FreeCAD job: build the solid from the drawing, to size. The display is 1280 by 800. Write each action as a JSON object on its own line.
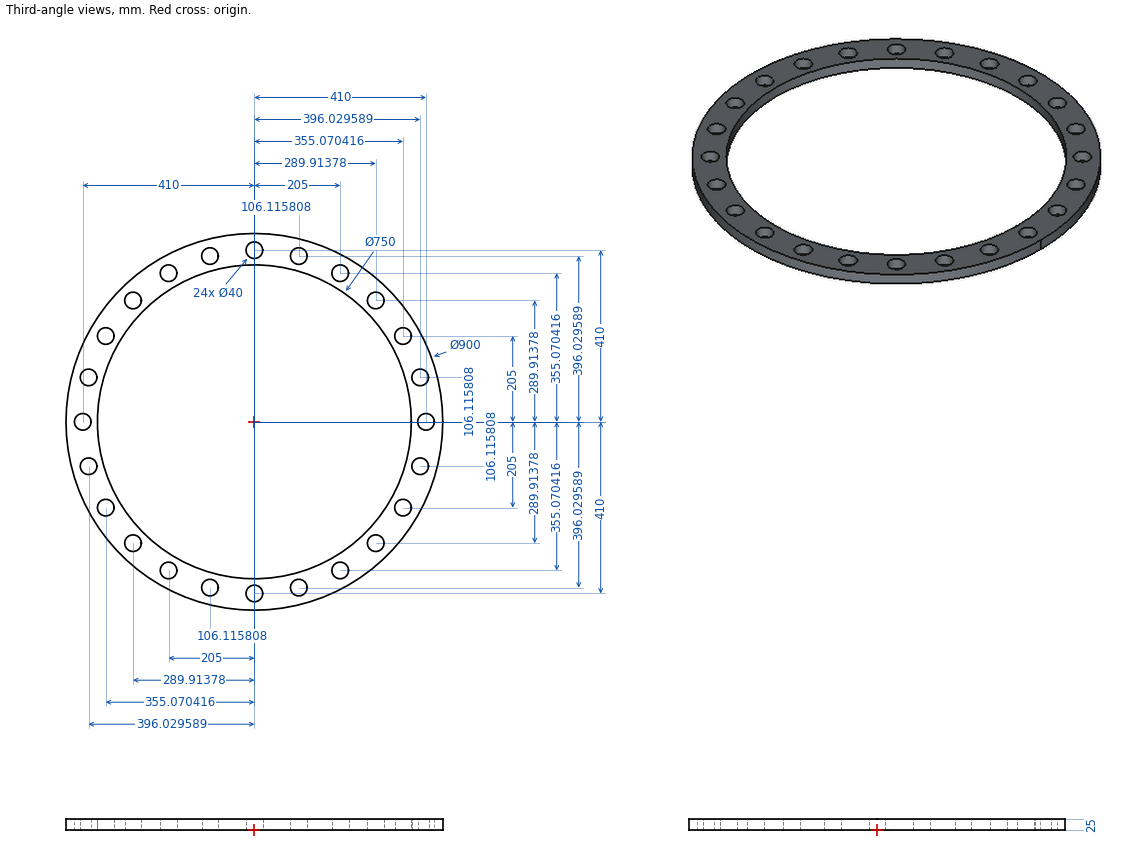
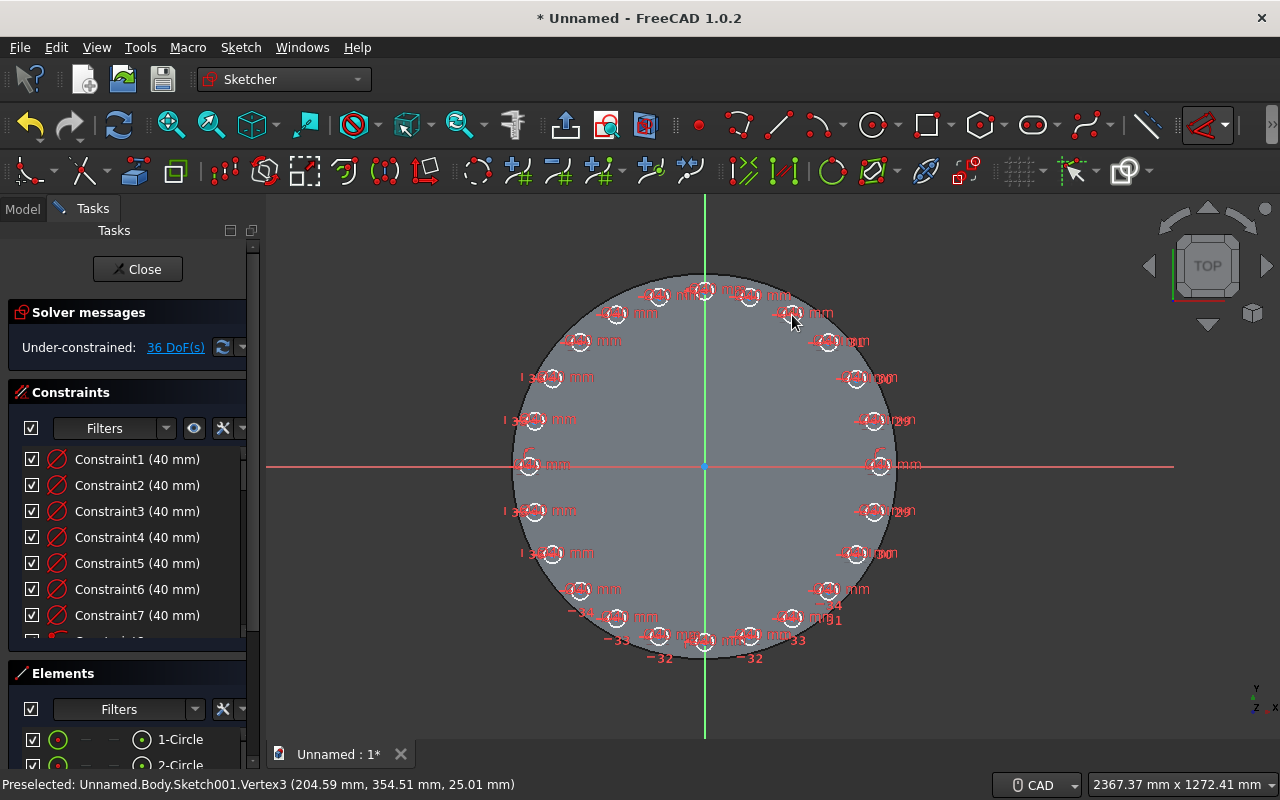
{"action": "left_click", "coordinate": [617, 315]}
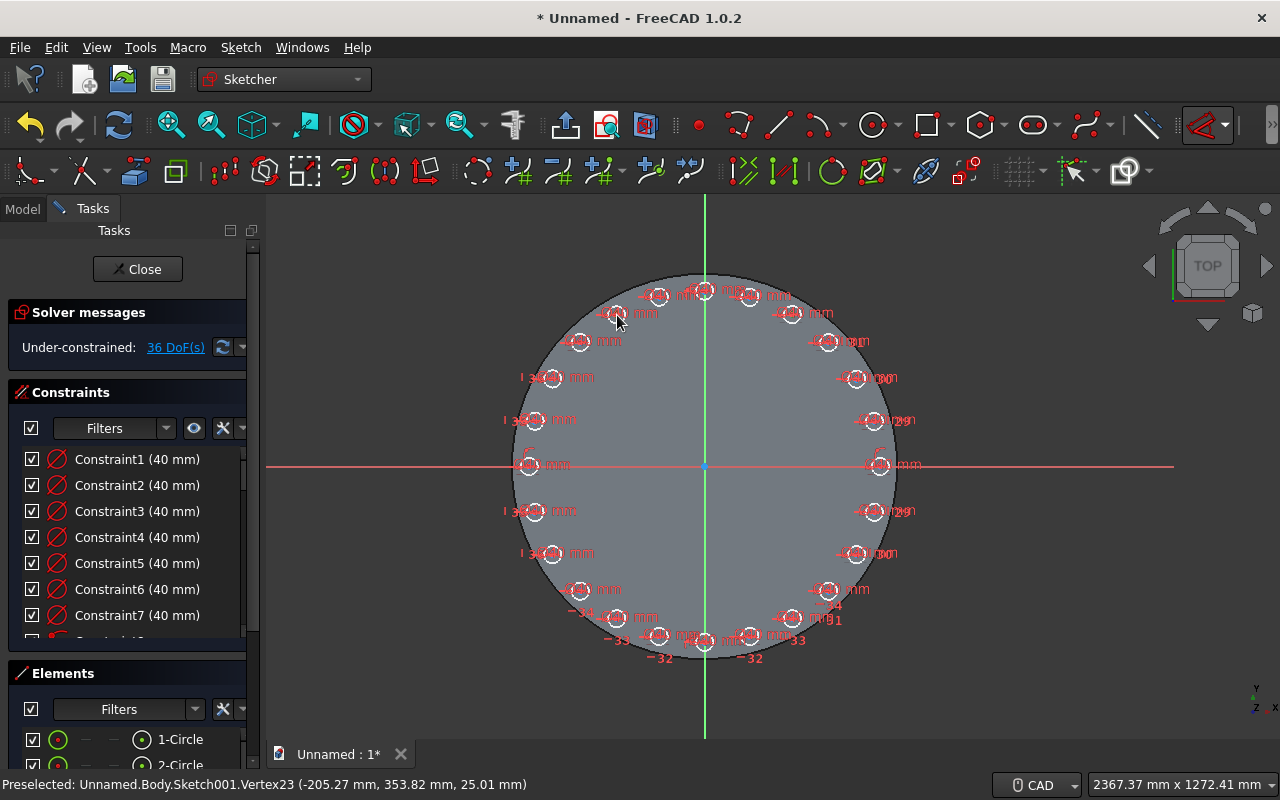
{"action": "key", "text": "h"}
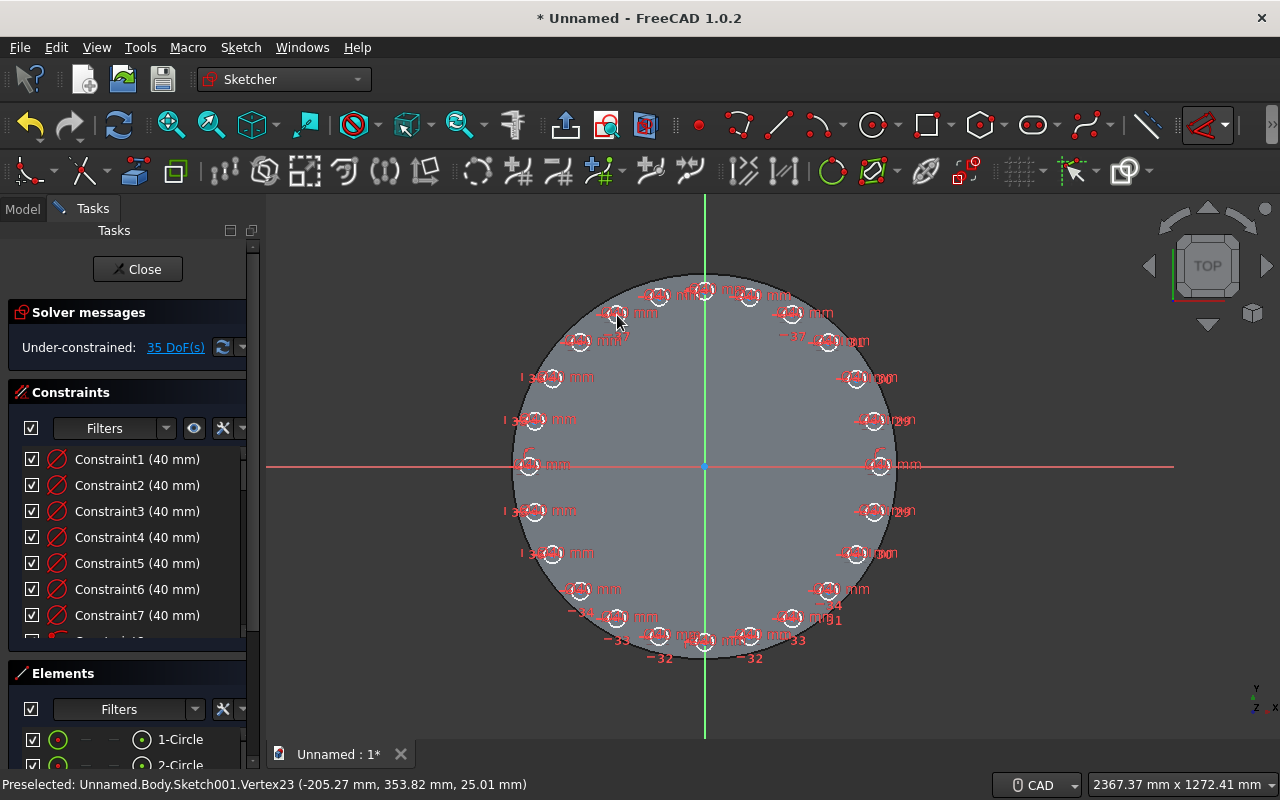
{"action": "left_click", "coordinate": [750, 297]}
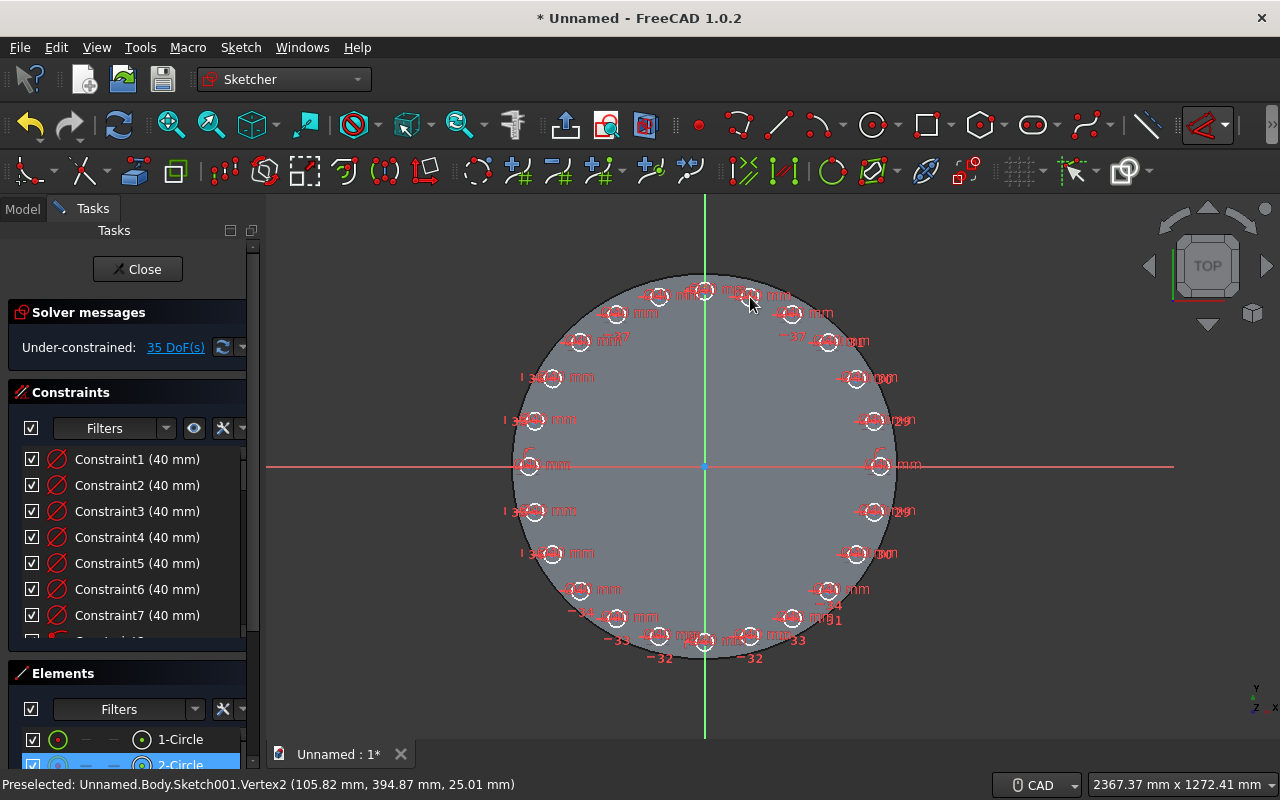
{"action": "left_click", "coordinate": [659, 297]}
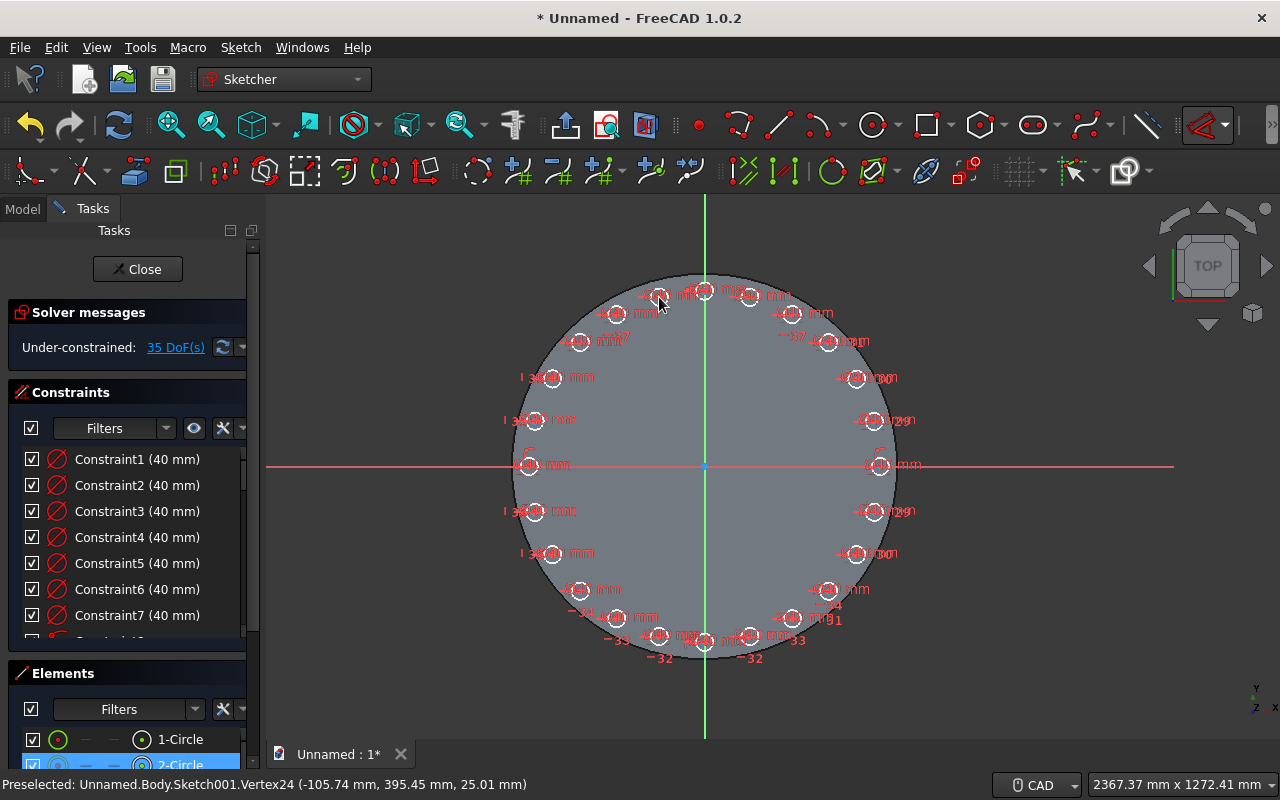
{"action": "key", "text": "h"}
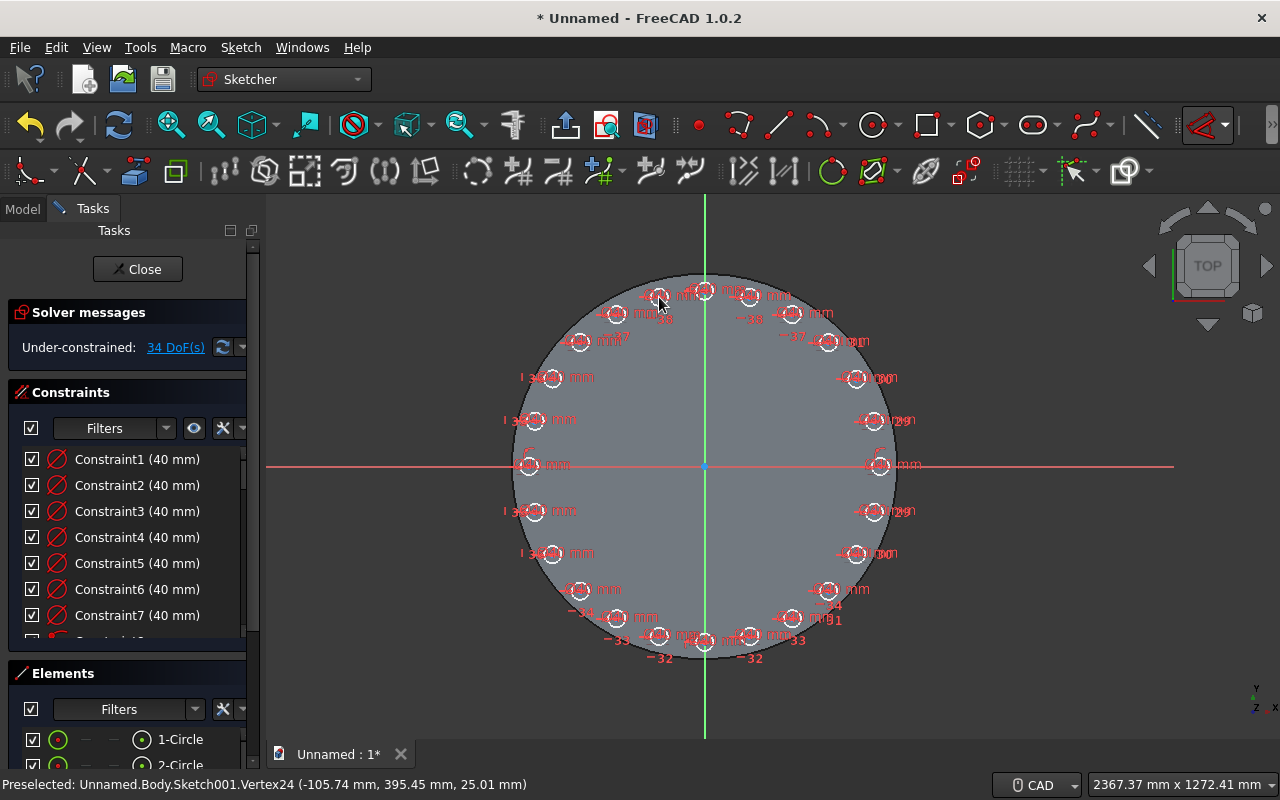
{"action": "left_click", "coordinate": [1202, 126]}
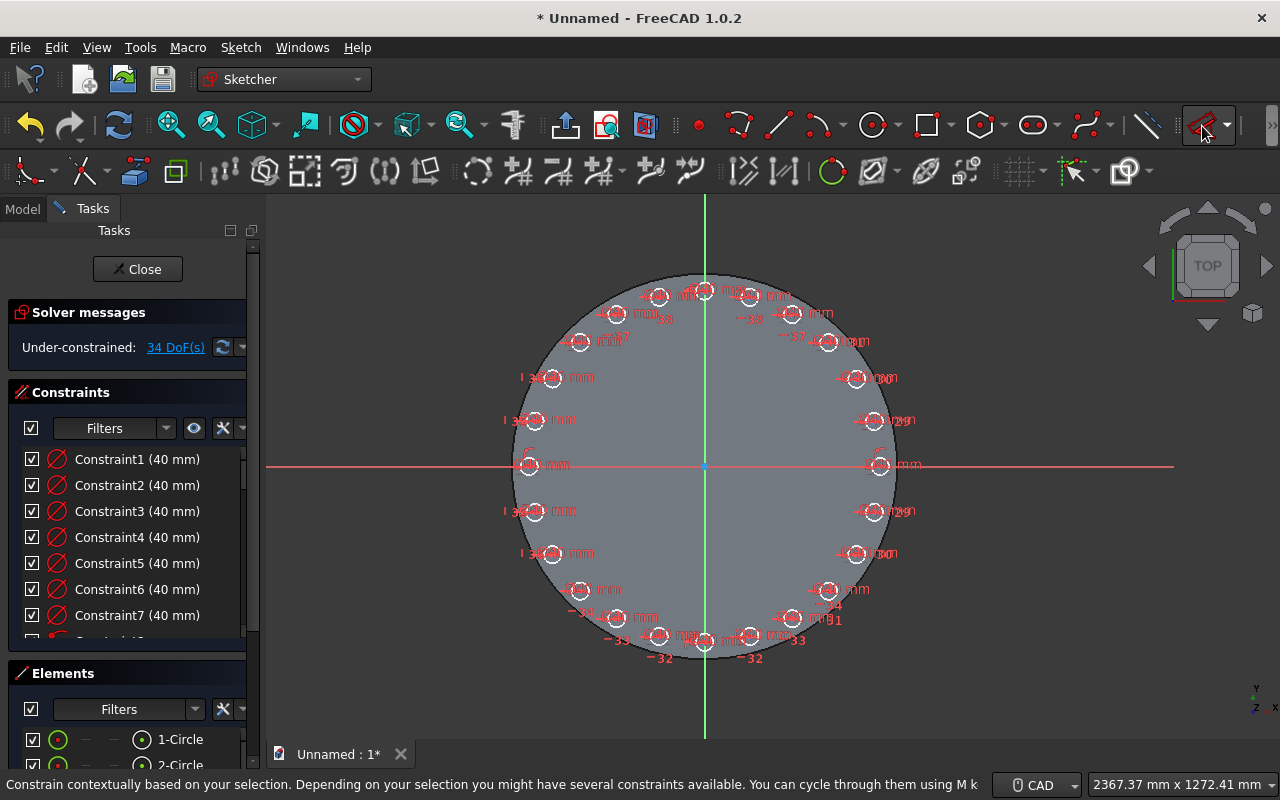
{"action": "left_click", "coordinate": [705, 291]}
{"action": "left_click", "coordinate": [739, 379]}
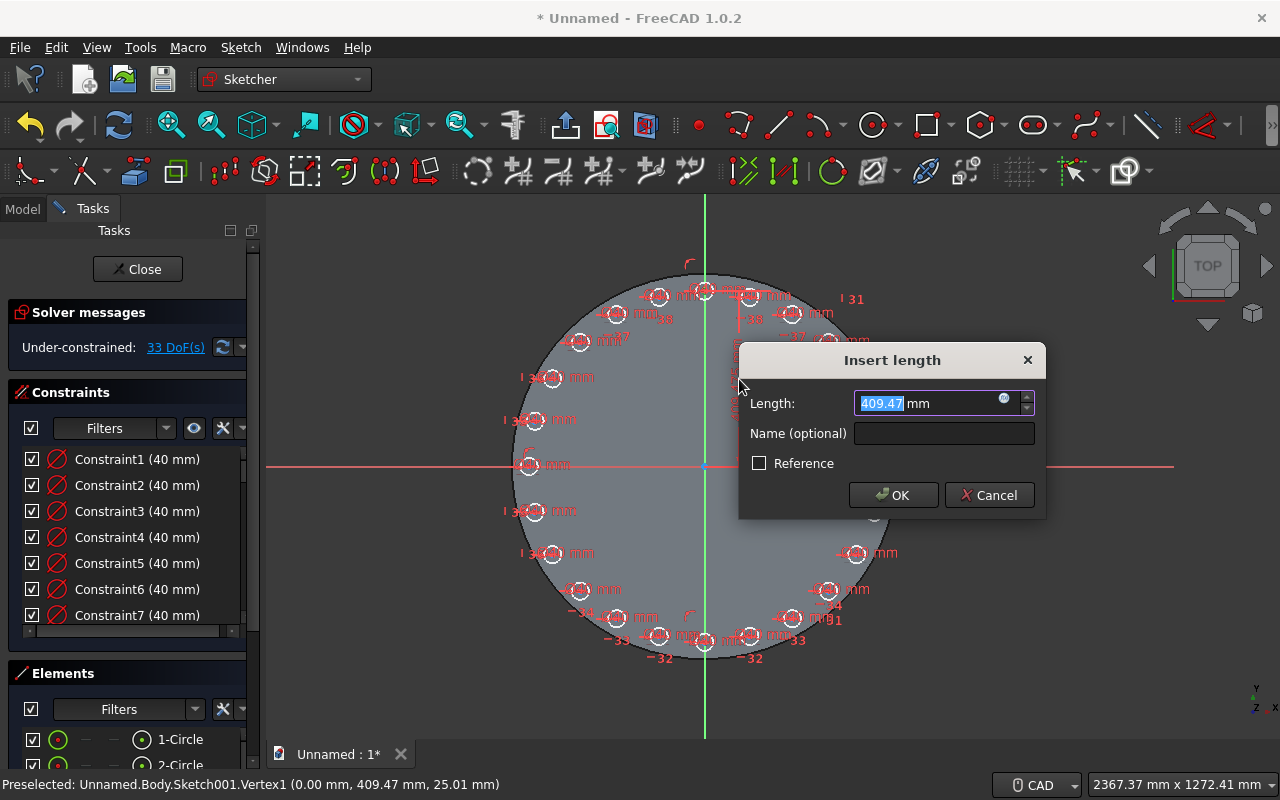
{"action": "type", "text": "410"}
{"action": "key", "text": "Return"}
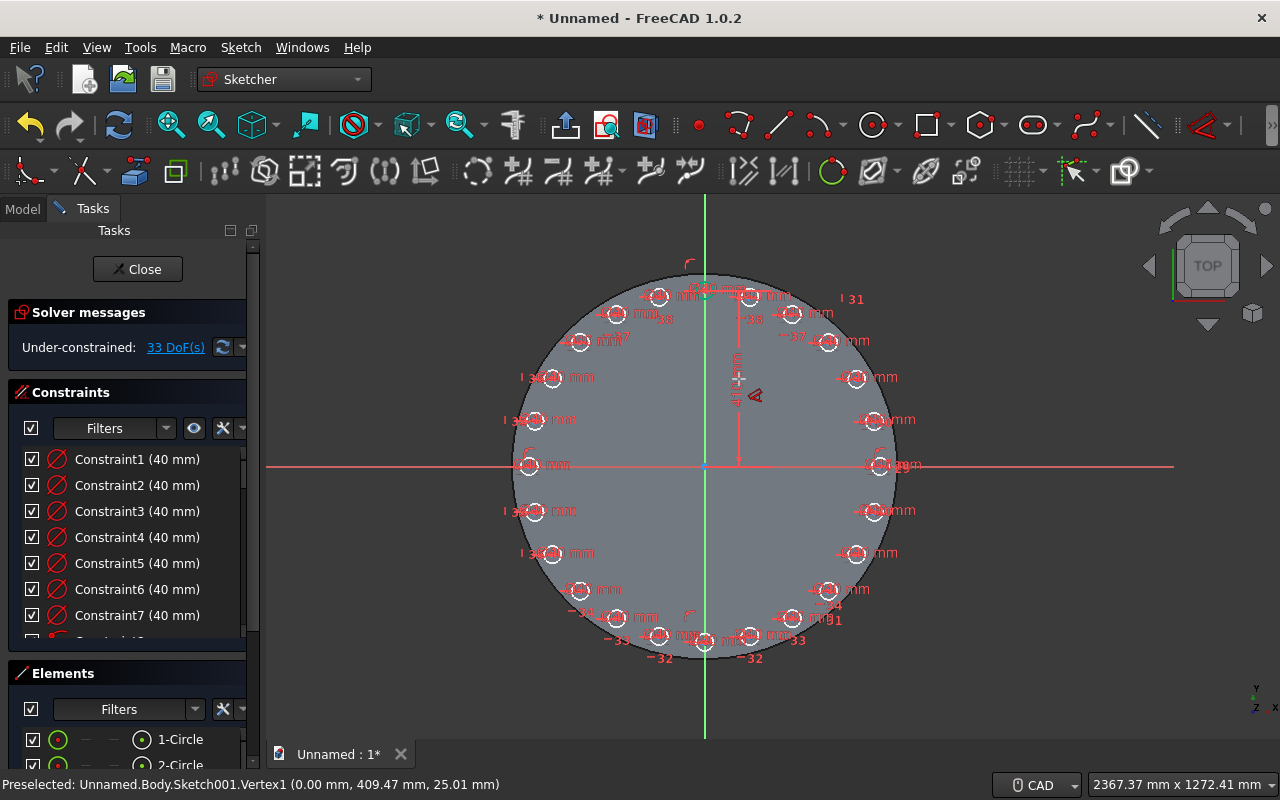
{"action": "left_click", "coordinate": [792, 315]}
{"action": "left_click", "coordinate": [728, 281]}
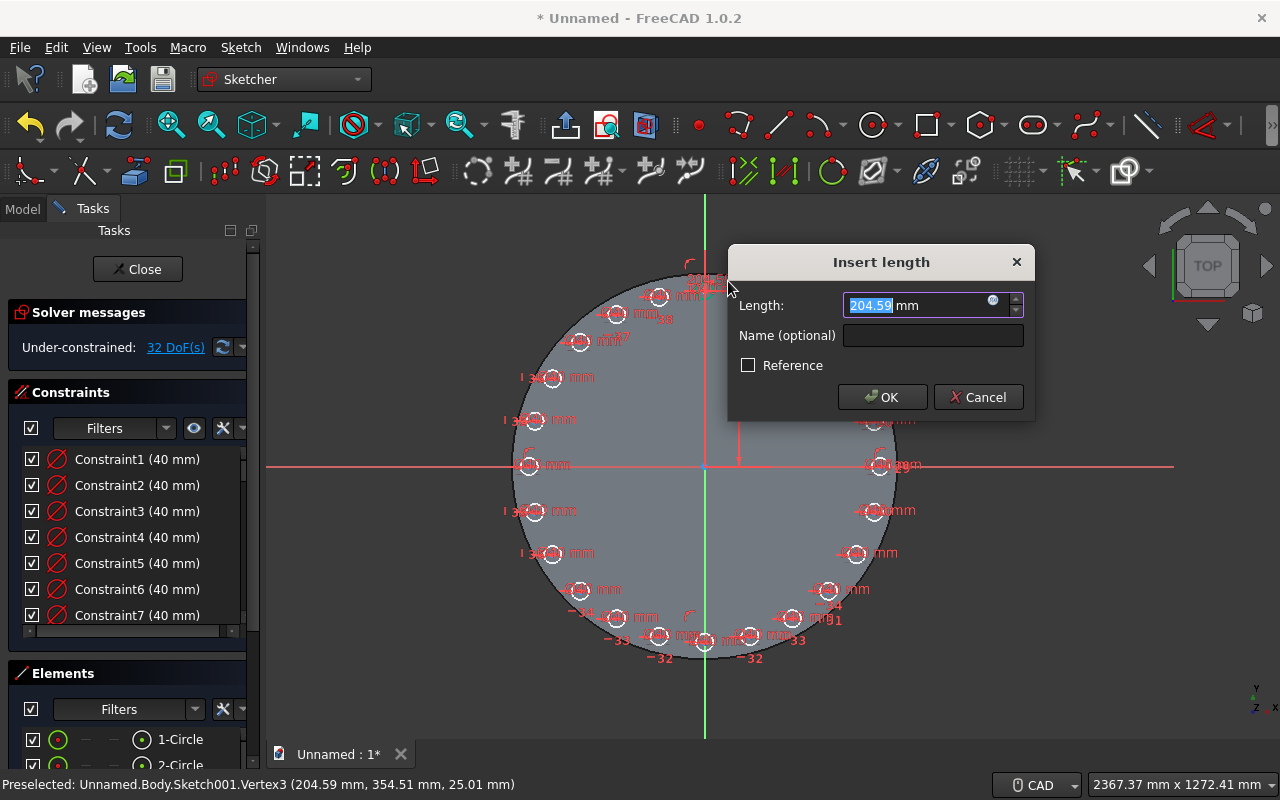
{"action": "type", "text": "205"}
{"action": "key", "text": "Return"}